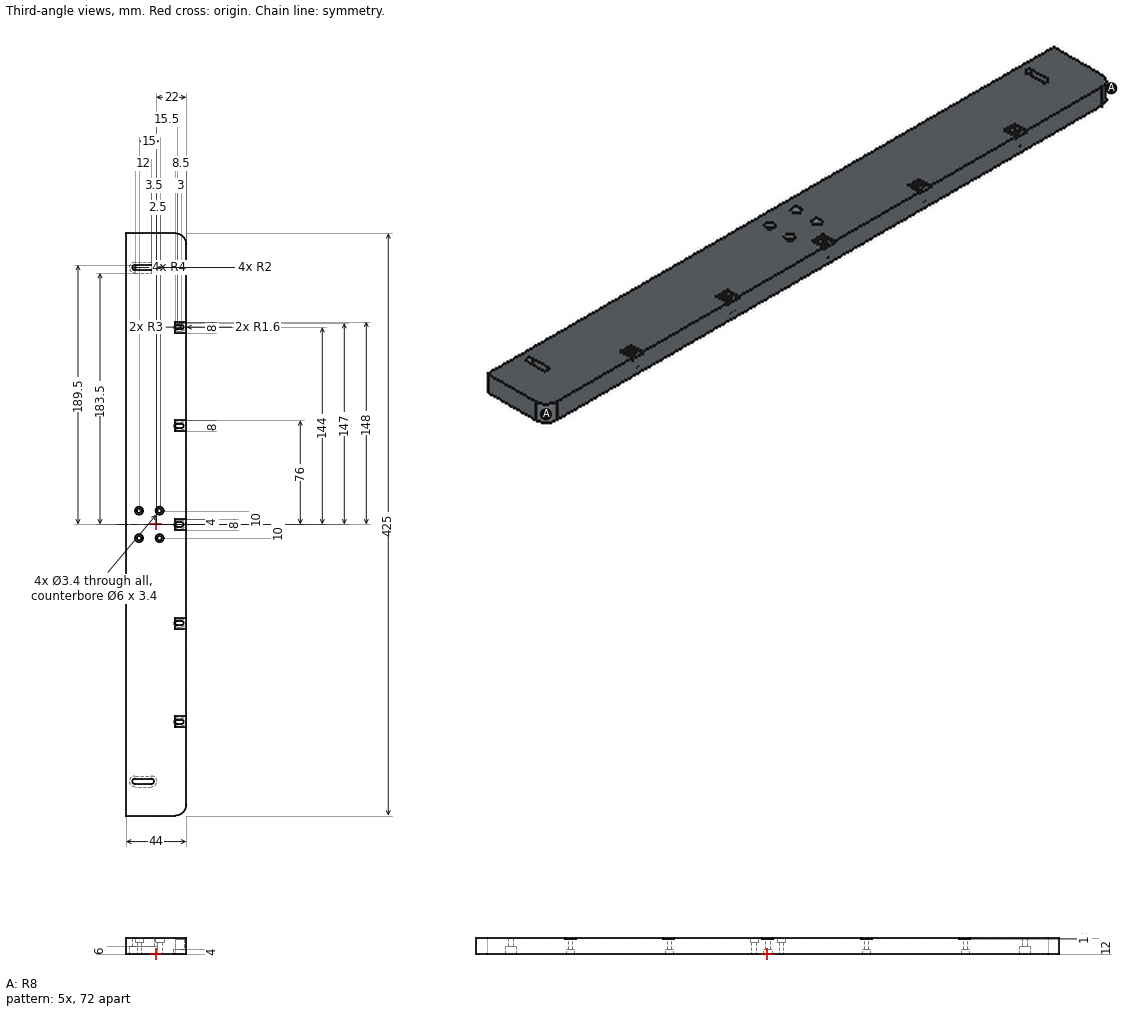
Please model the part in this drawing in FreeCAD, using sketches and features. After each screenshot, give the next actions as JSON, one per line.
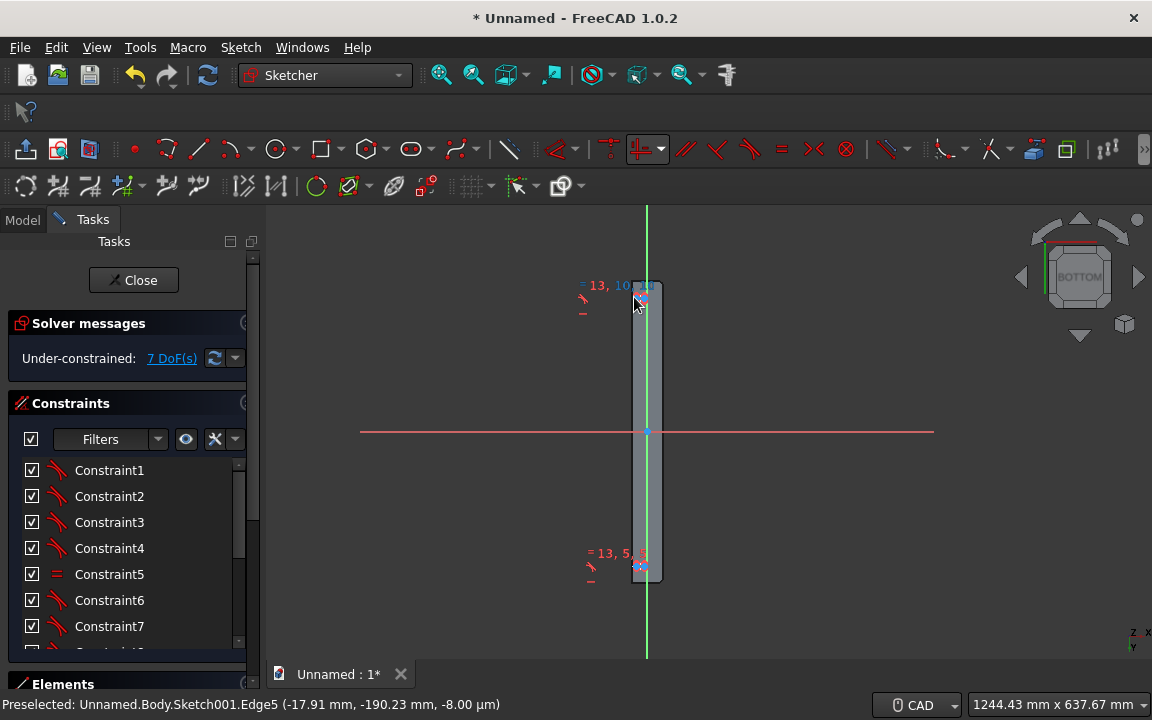
{"action": "scroll", "coordinate": [636, 566], "scroll_direction": "up", "scroll_amount": 8}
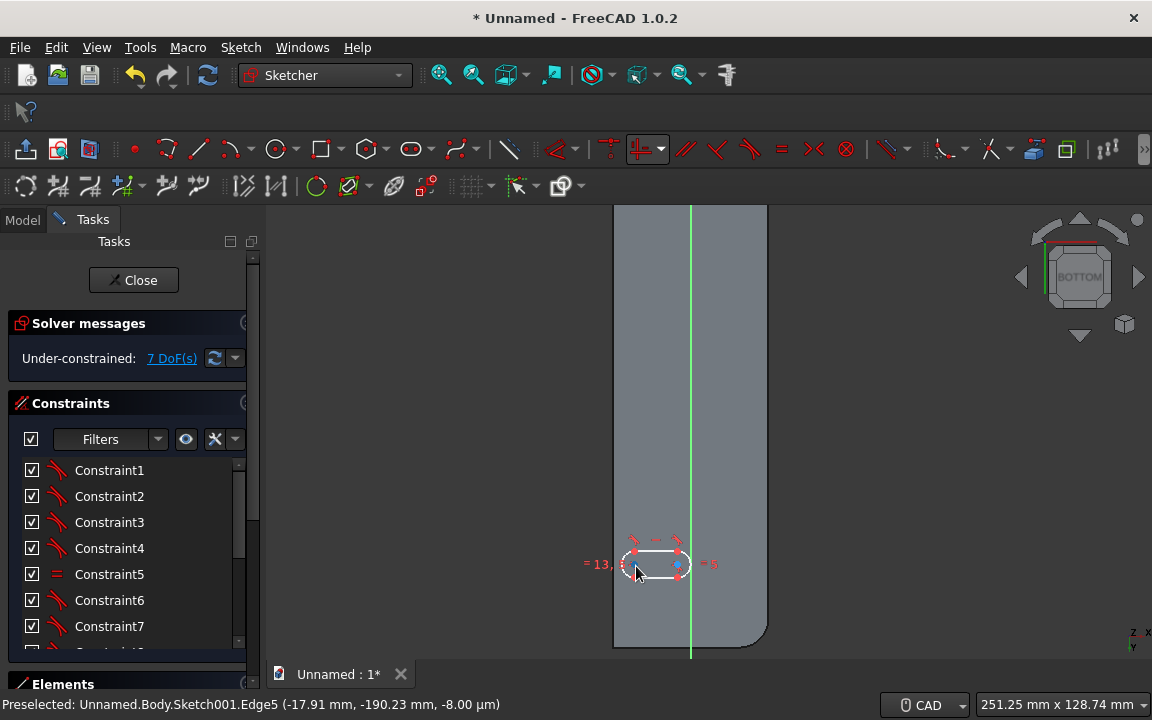
{"action": "left_click", "coordinate": [635, 564]}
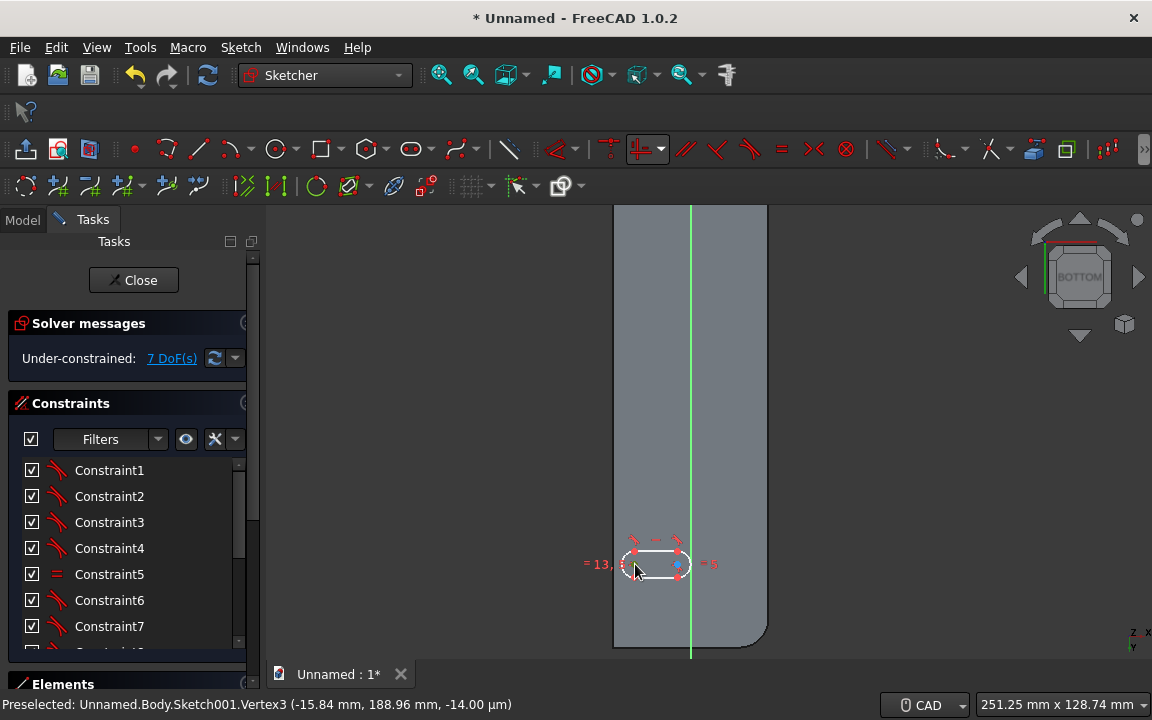
{"action": "scroll", "coordinate": [636, 567], "scroll_direction": "down", "scroll_amount": 8}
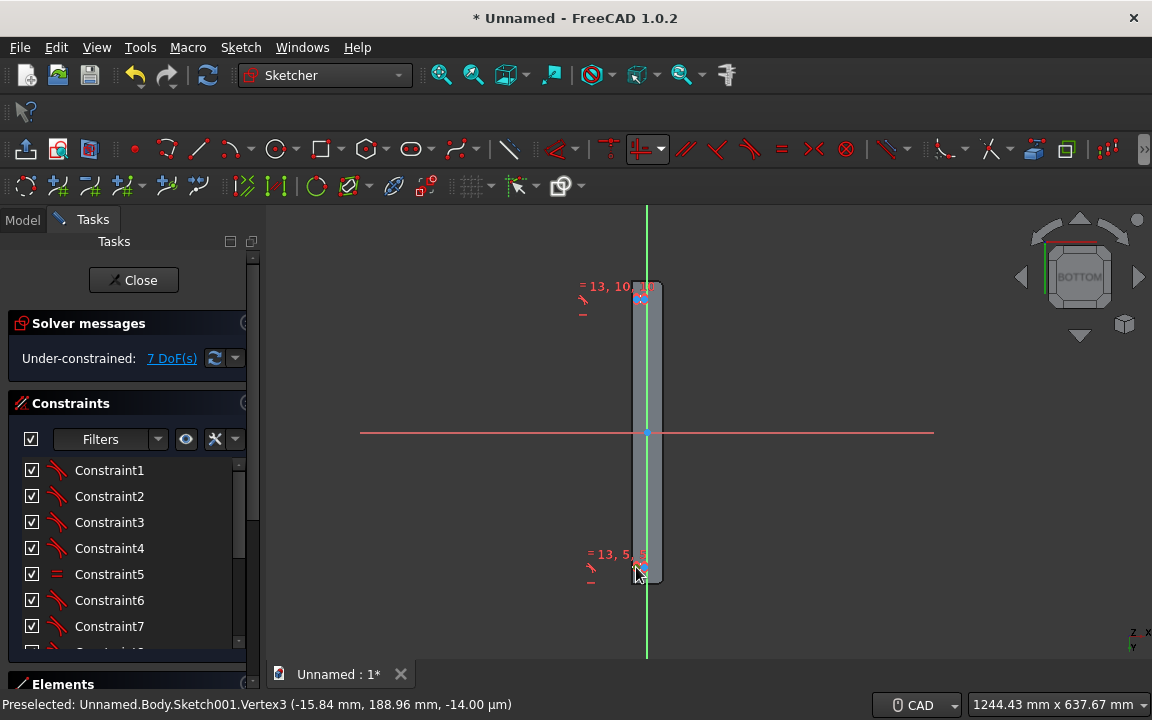
{"action": "scroll", "coordinate": [636, 299], "scroll_direction": "up", "scroll_amount": 8}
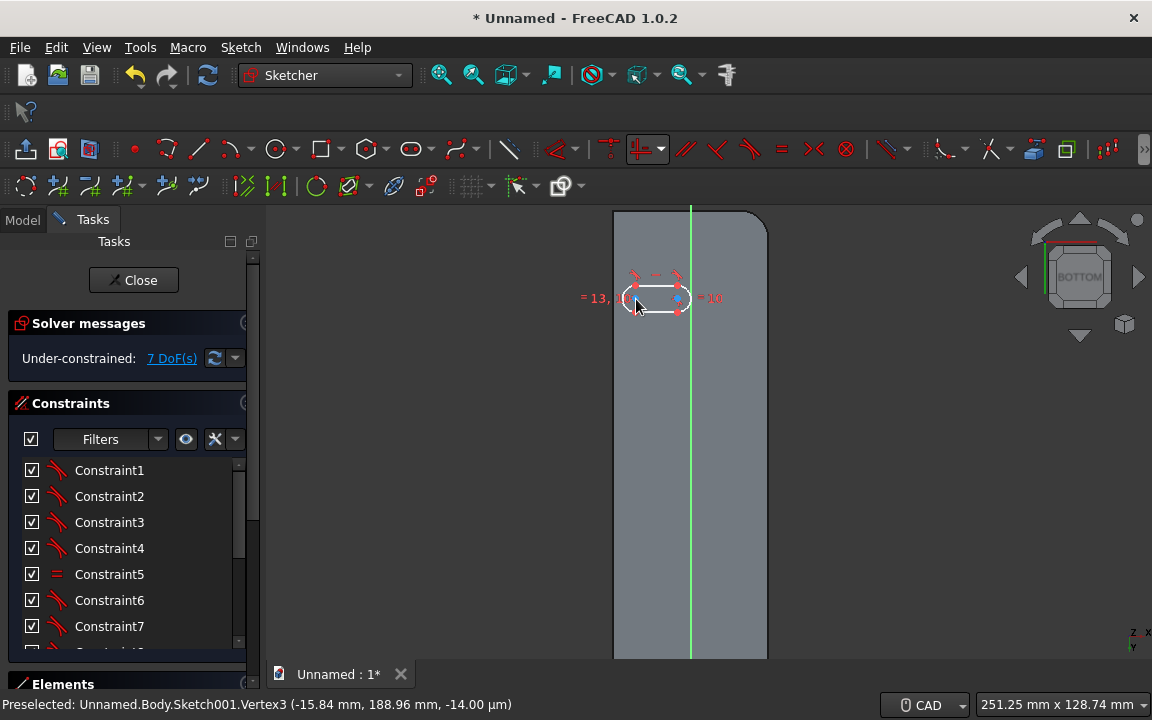
{"action": "left_click", "coordinate": [636, 299]}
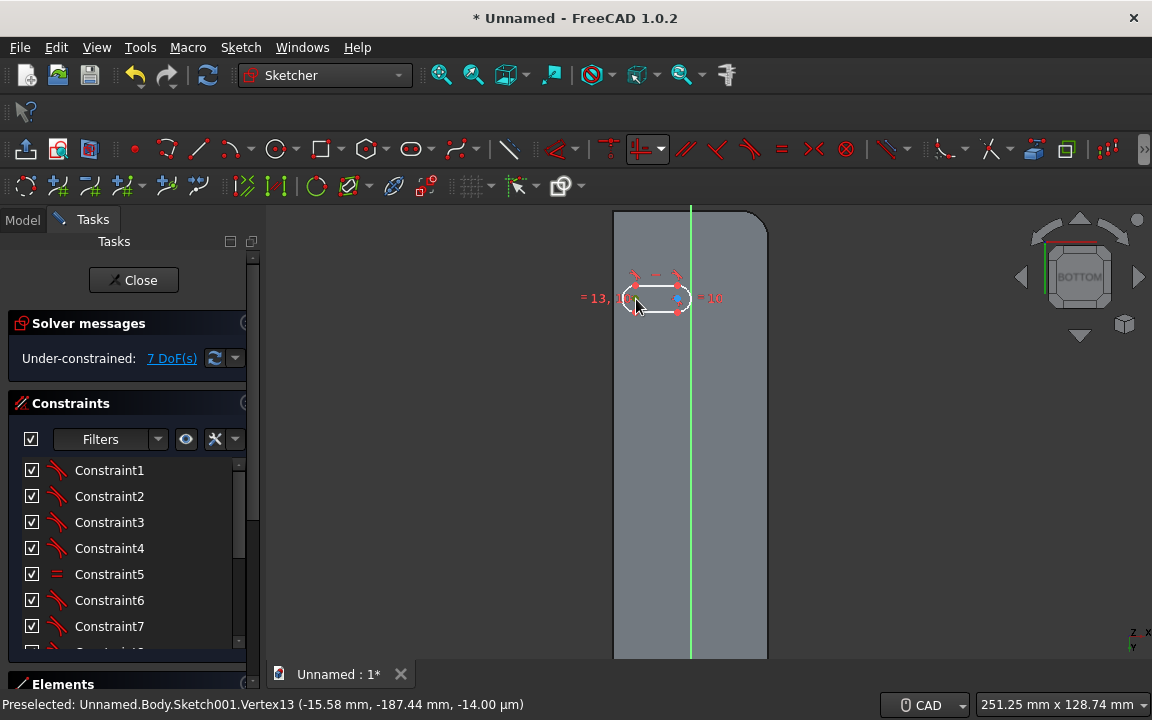
{"action": "scroll", "coordinate": [636, 298], "scroll_direction": "down", "scroll_amount": 8}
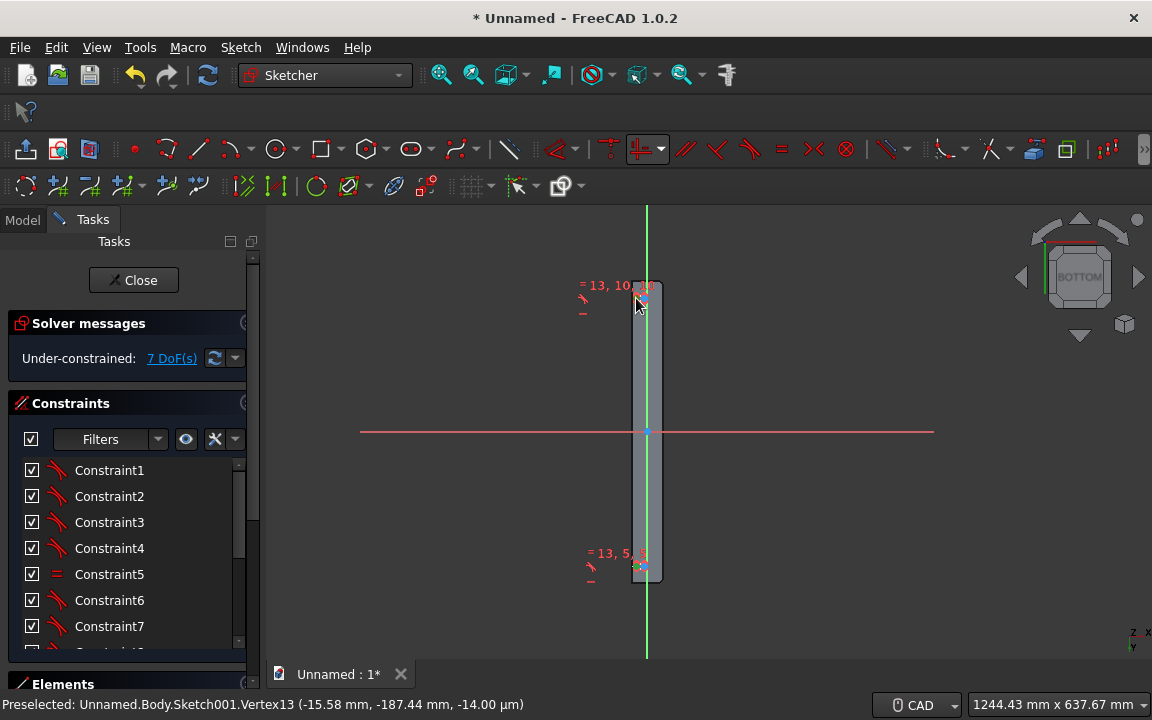
{"action": "left_click", "coordinate": [393, 432]}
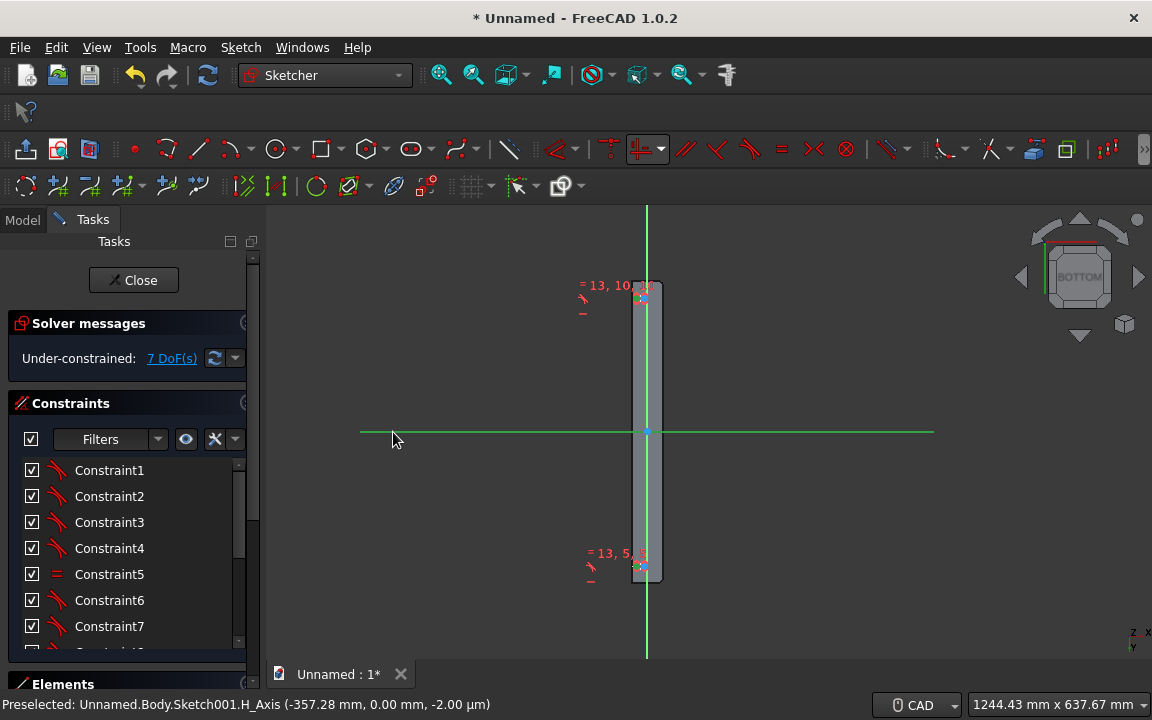
{"action": "left_click", "coordinate": [814, 150]}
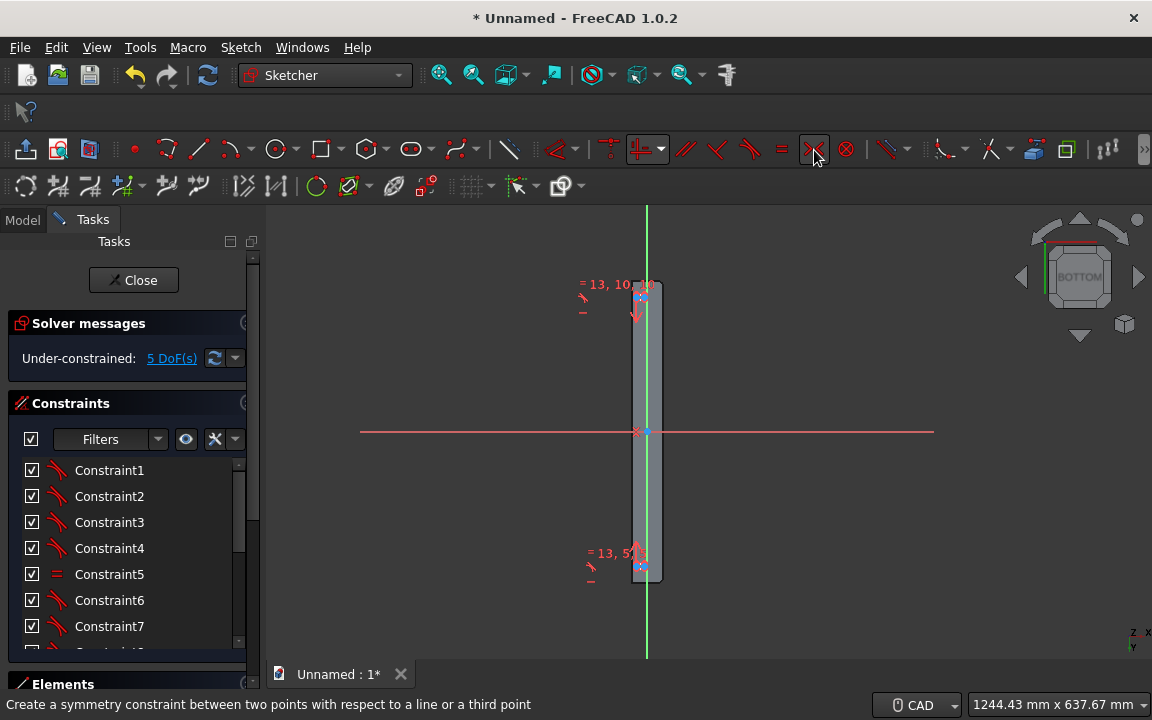
{"action": "scroll", "coordinate": [634, 566], "scroll_direction": "up", "scroll_amount": 14}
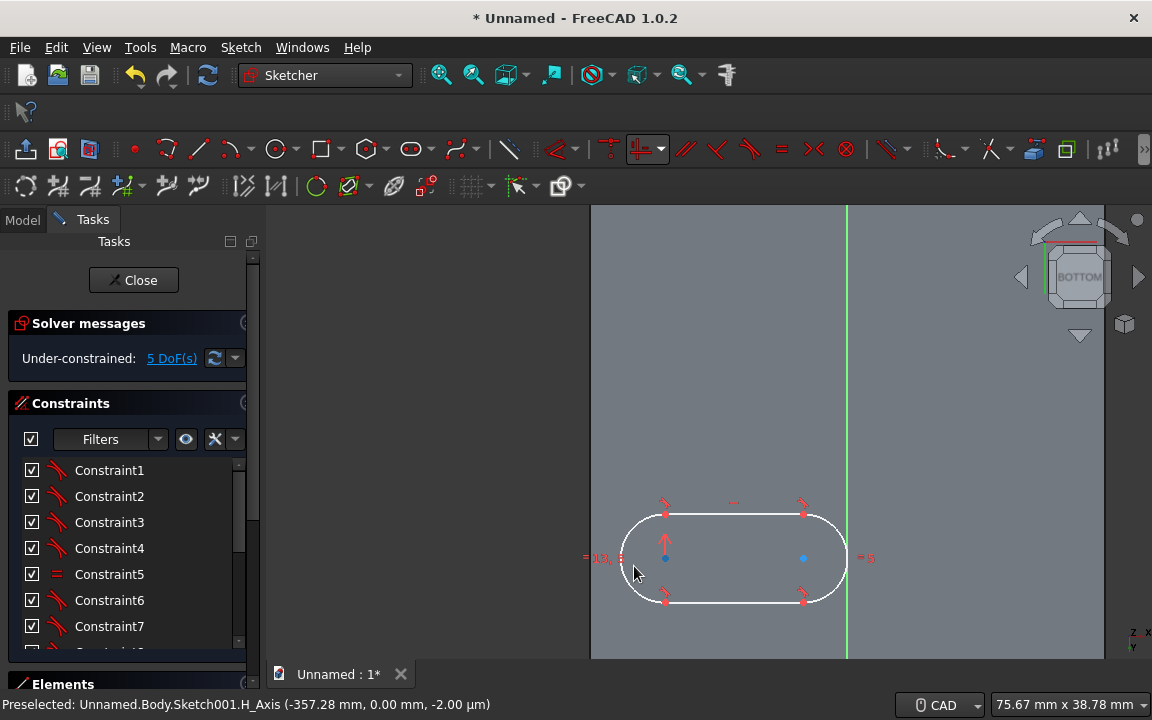
{"action": "left_click", "coordinate": [629, 584]}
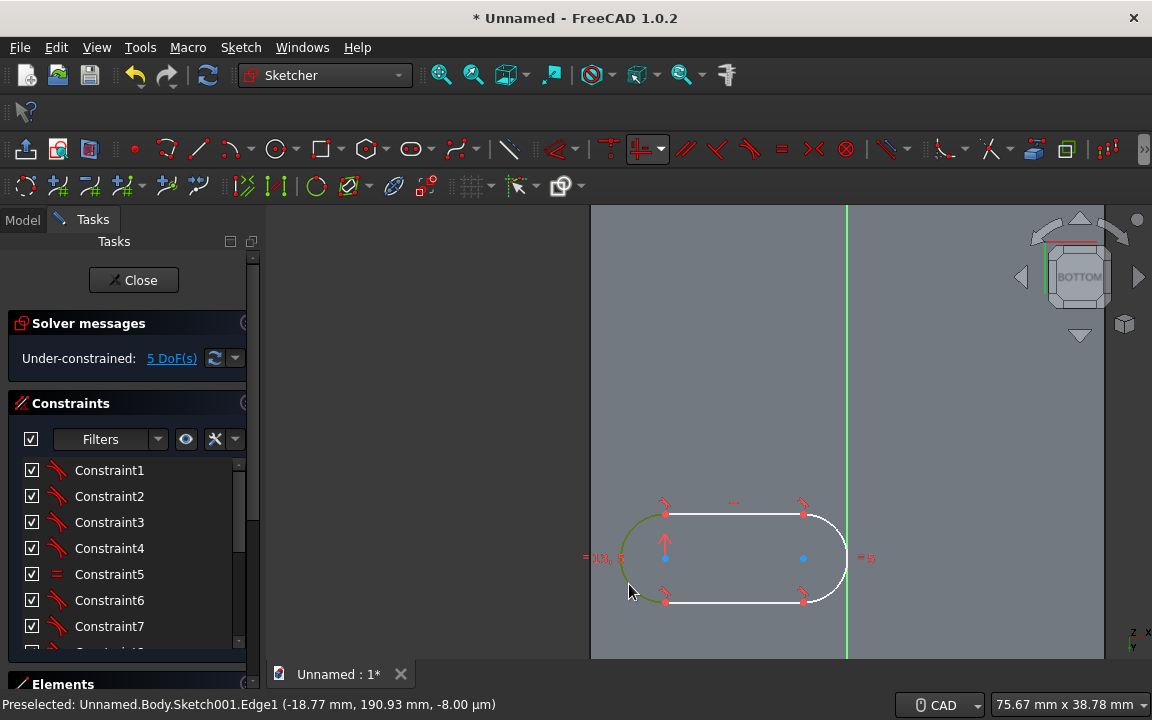
{"action": "left_click", "coordinate": [578, 150]}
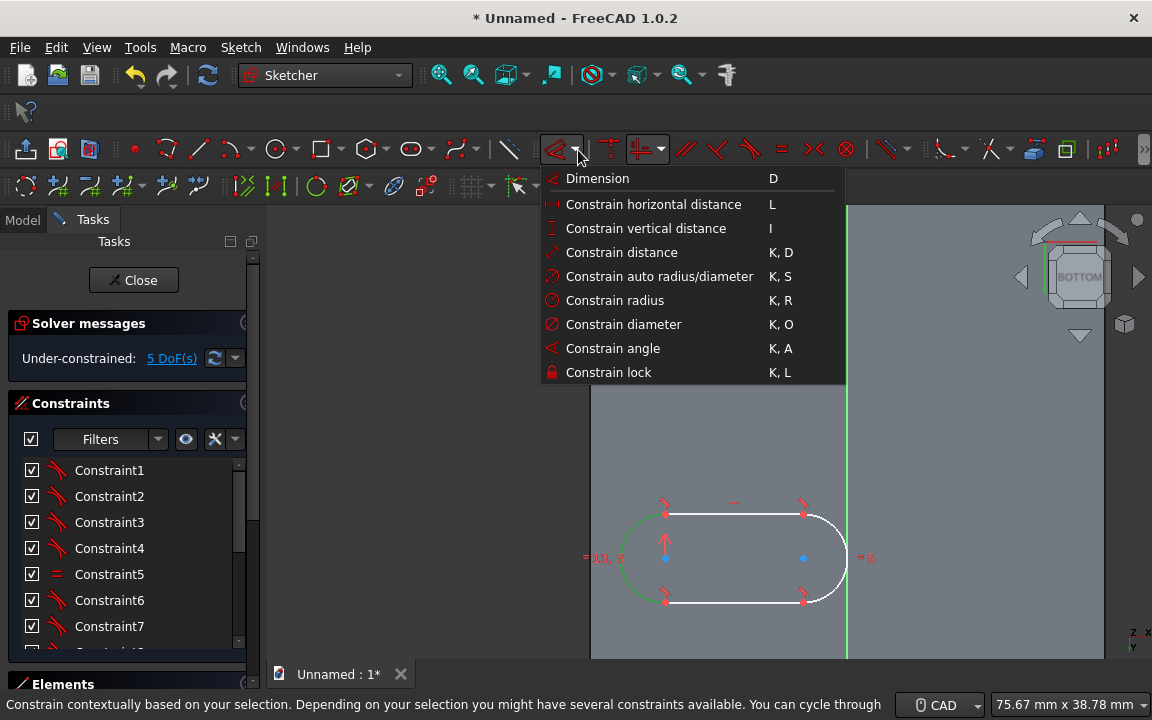
{"action": "left_click", "coordinate": [693, 300]}